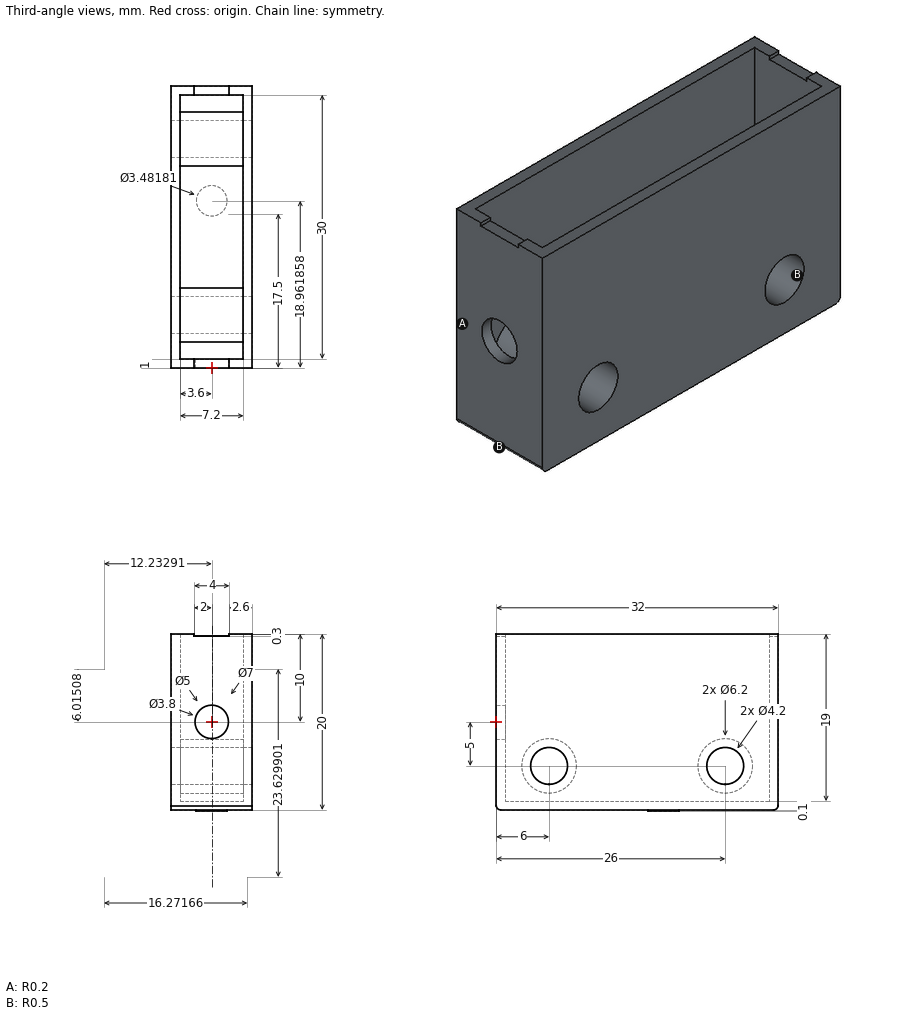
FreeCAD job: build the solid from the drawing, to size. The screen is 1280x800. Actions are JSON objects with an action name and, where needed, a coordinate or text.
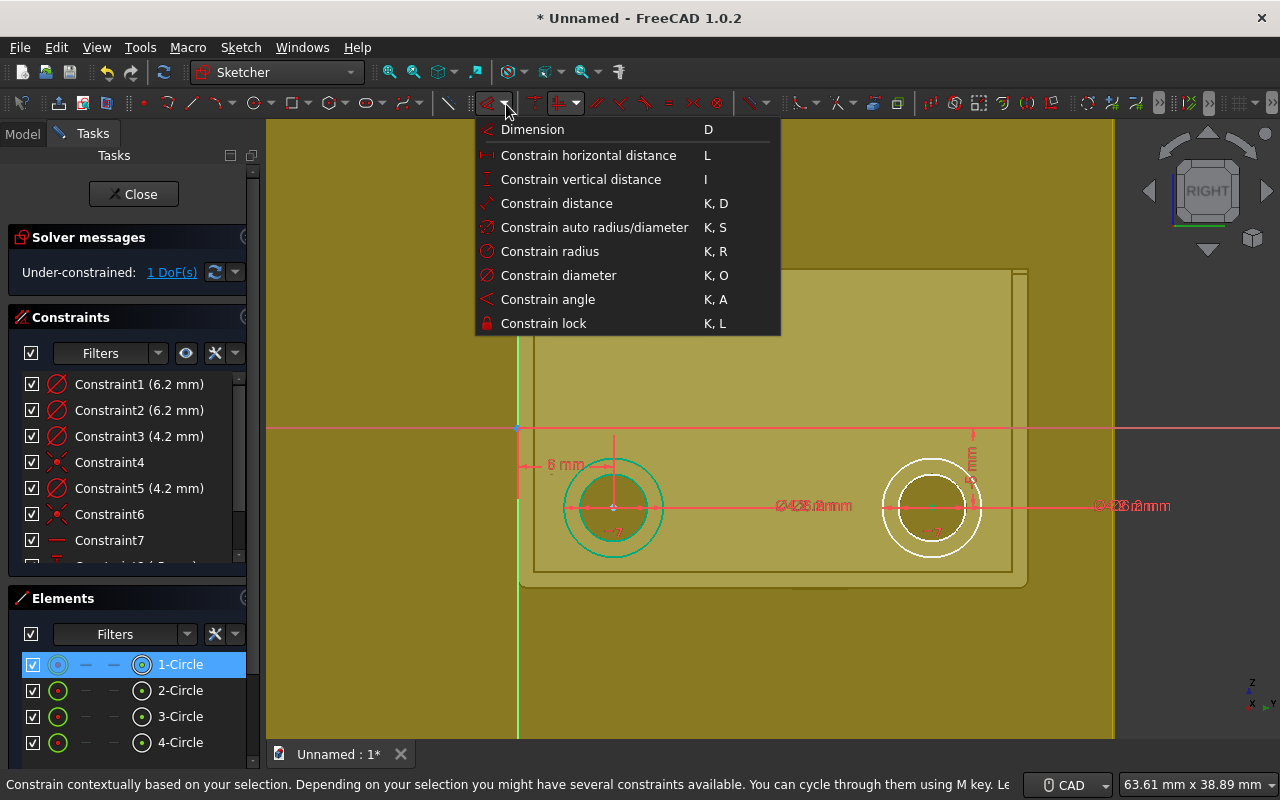
{"action": "left_click", "coordinate": [628, 155]}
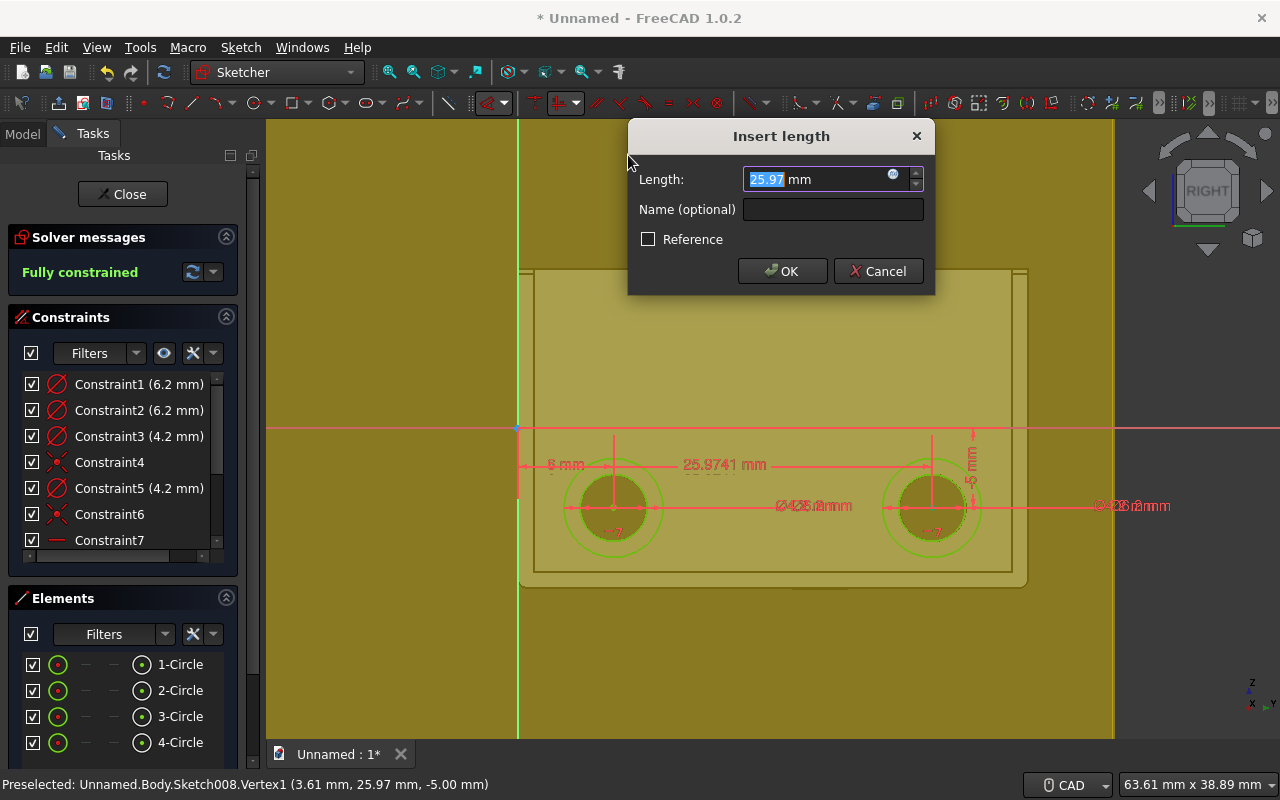
{"action": "type", "text": "26"}
{"action": "key", "text": "Return"}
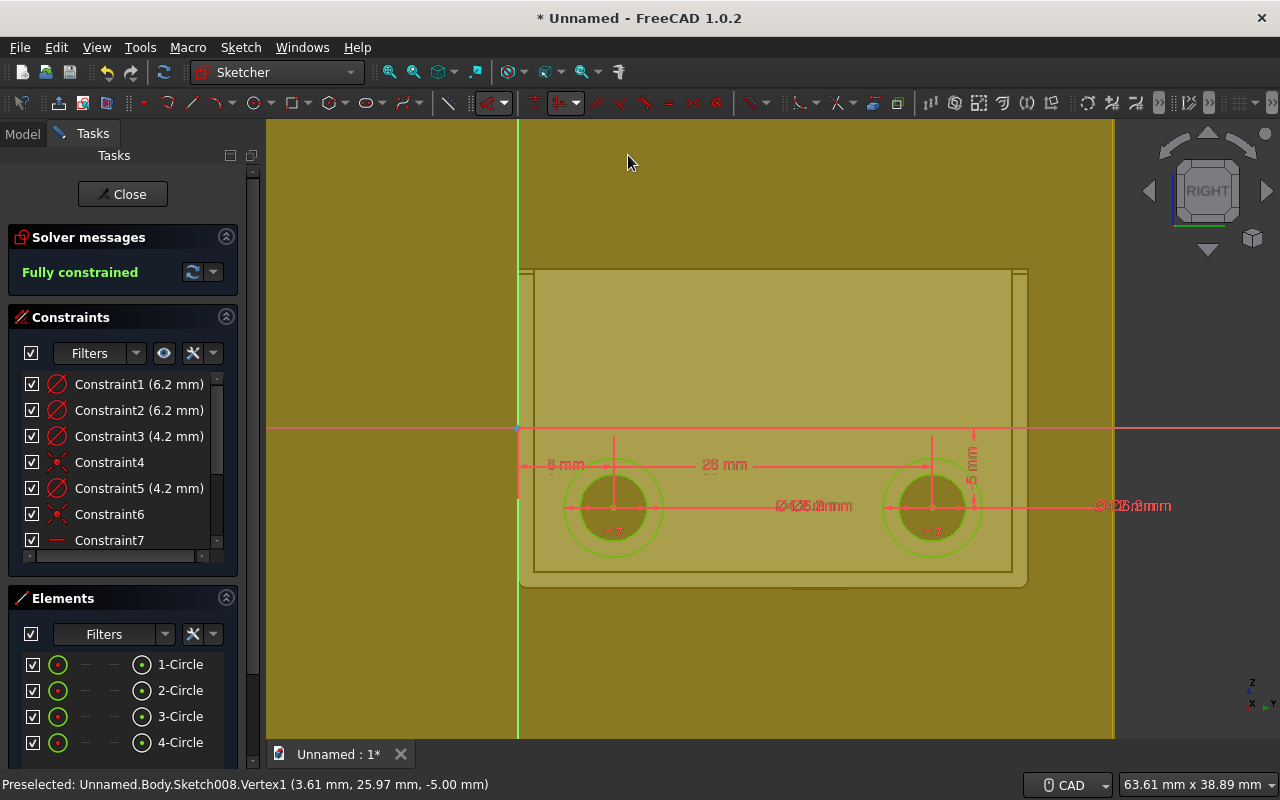
{"action": "left_click", "coordinate": [123, 194]}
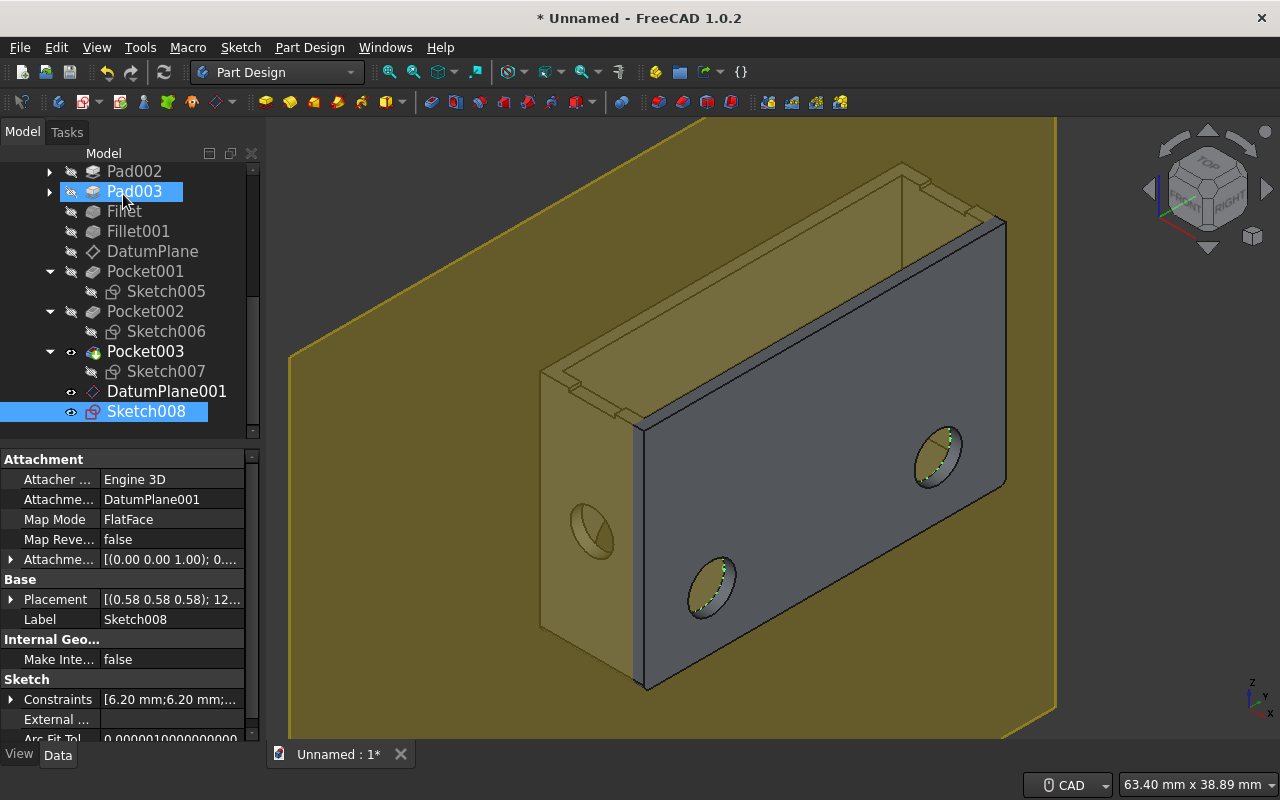
{"action": "left_click", "coordinate": [266, 102]}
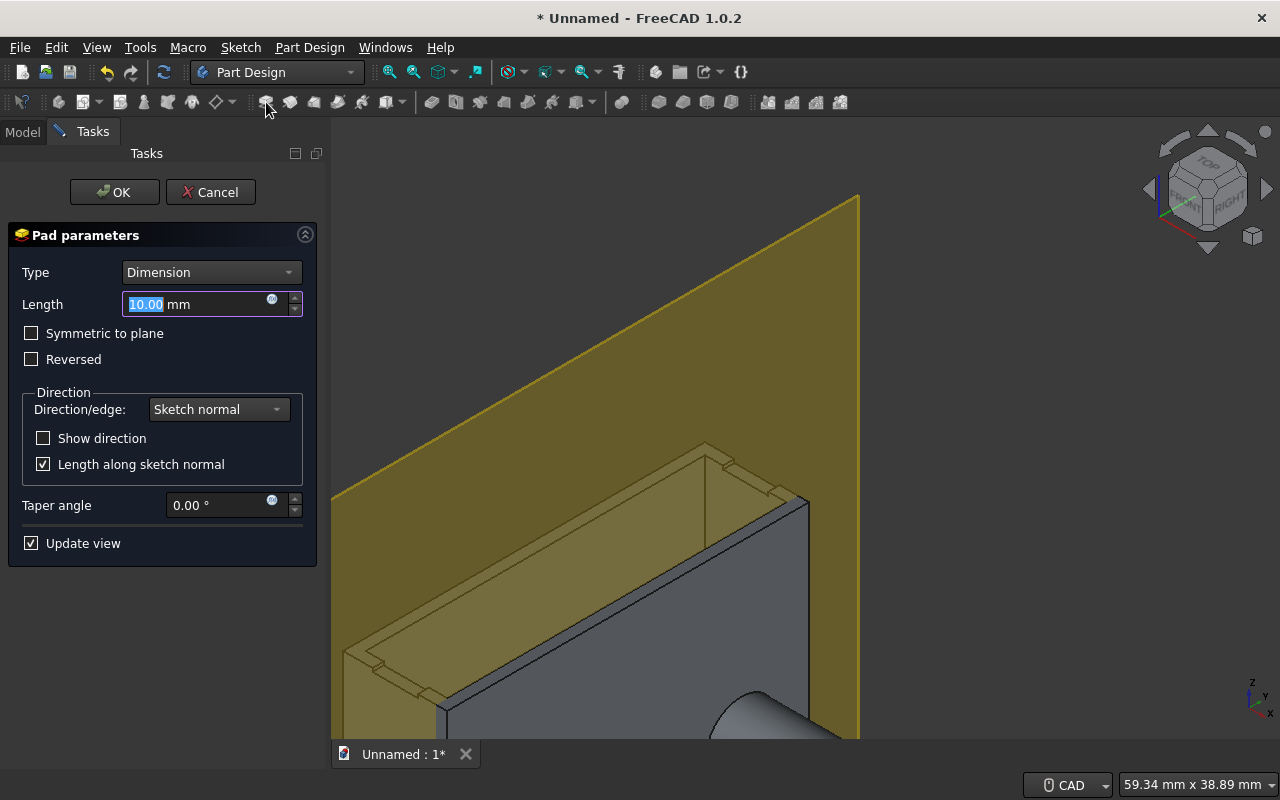
{"action": "type", "text": "7.2"}
{"action": "key", "text": "Tab"}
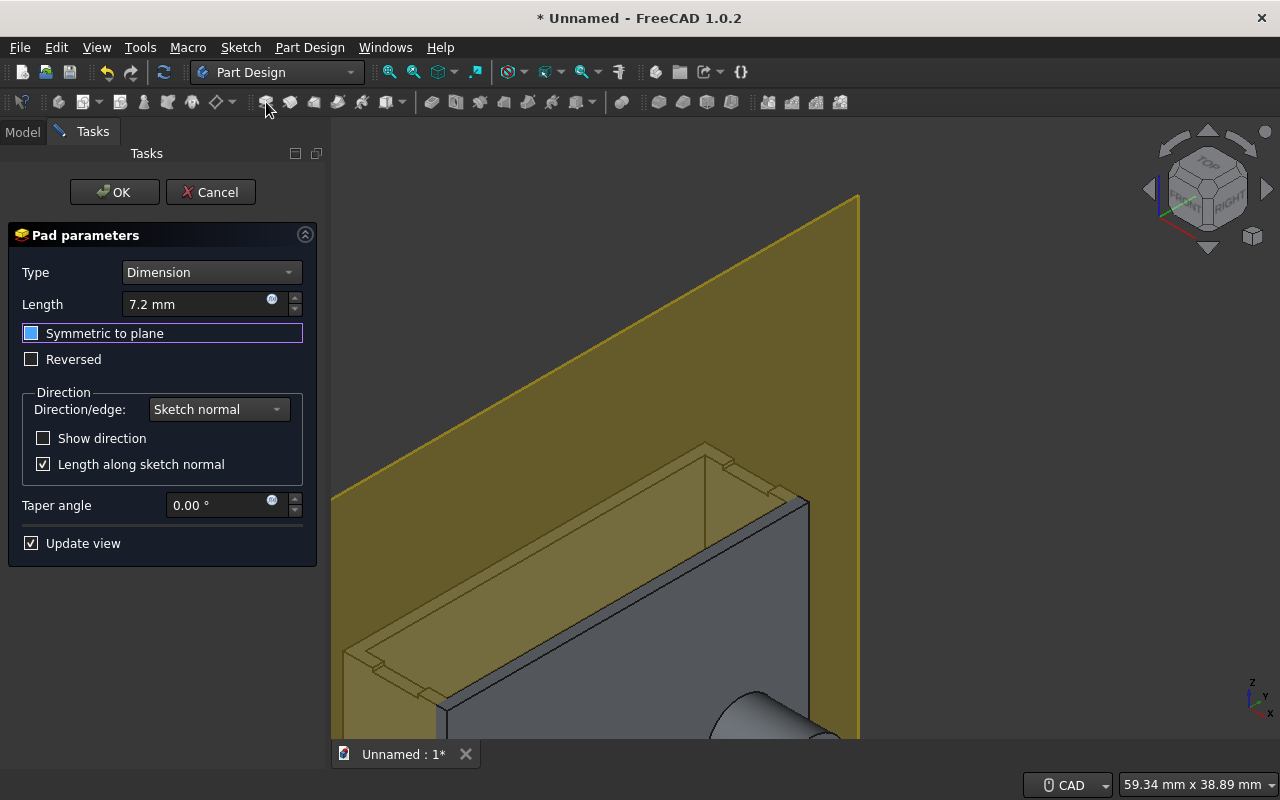
{"action": "left_click", "coordinate": [30, 359]}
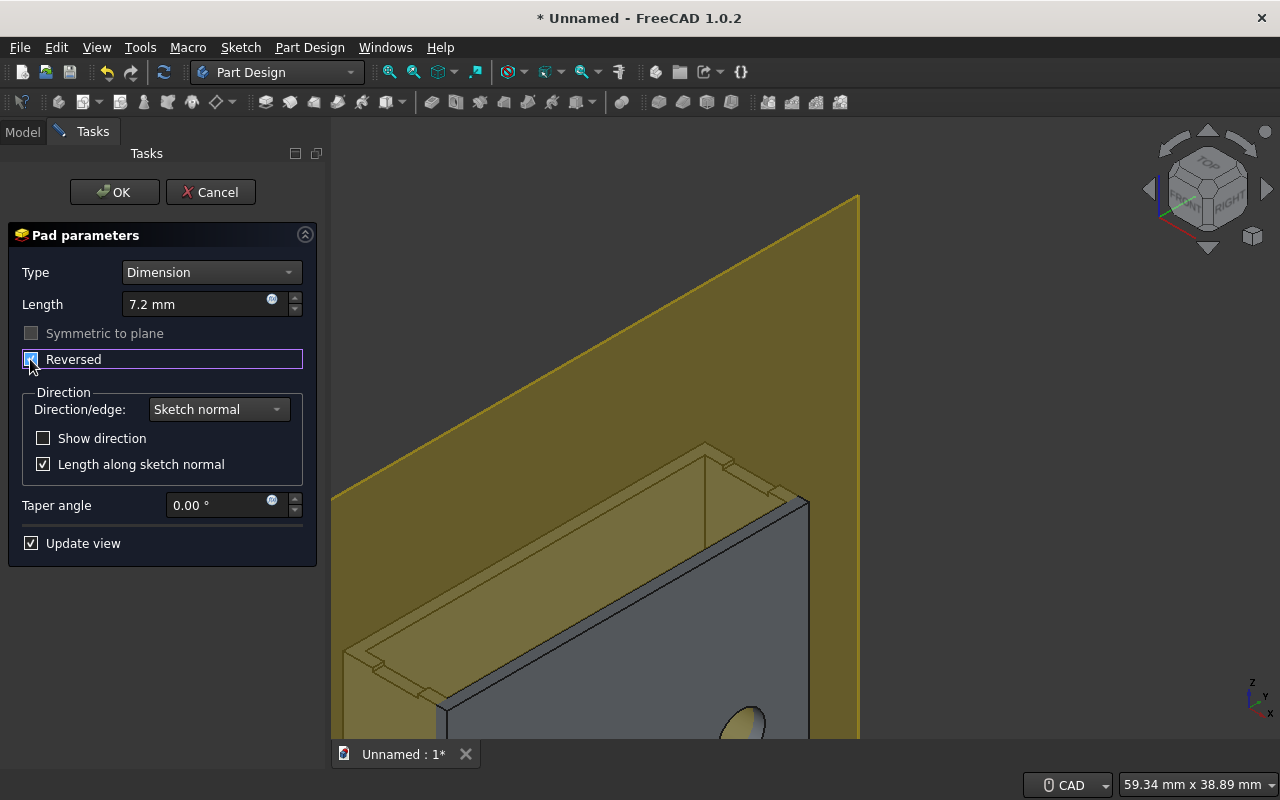
{"action": "left_click", "coordinate": [115, 192]}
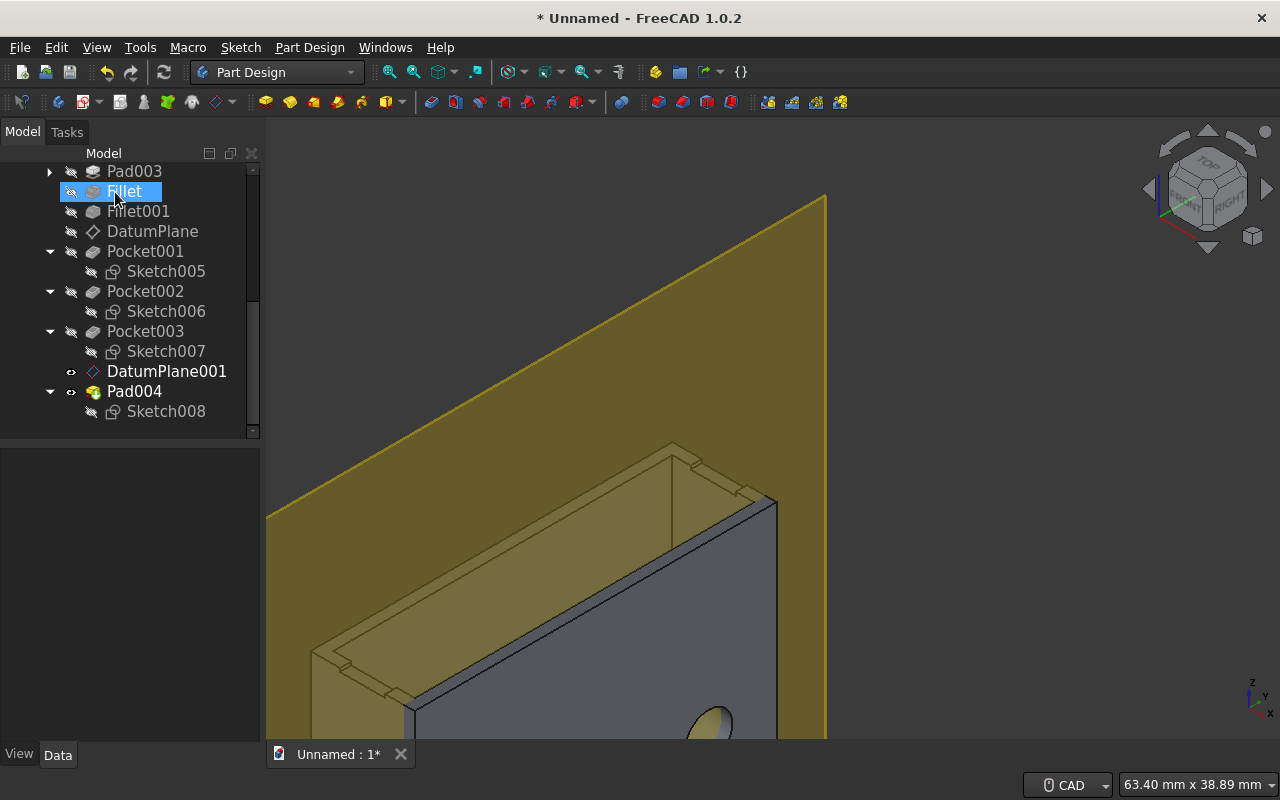
{"action": "left_click", "coordinate": [116, 372]}
{"action": "key", "text": "space"}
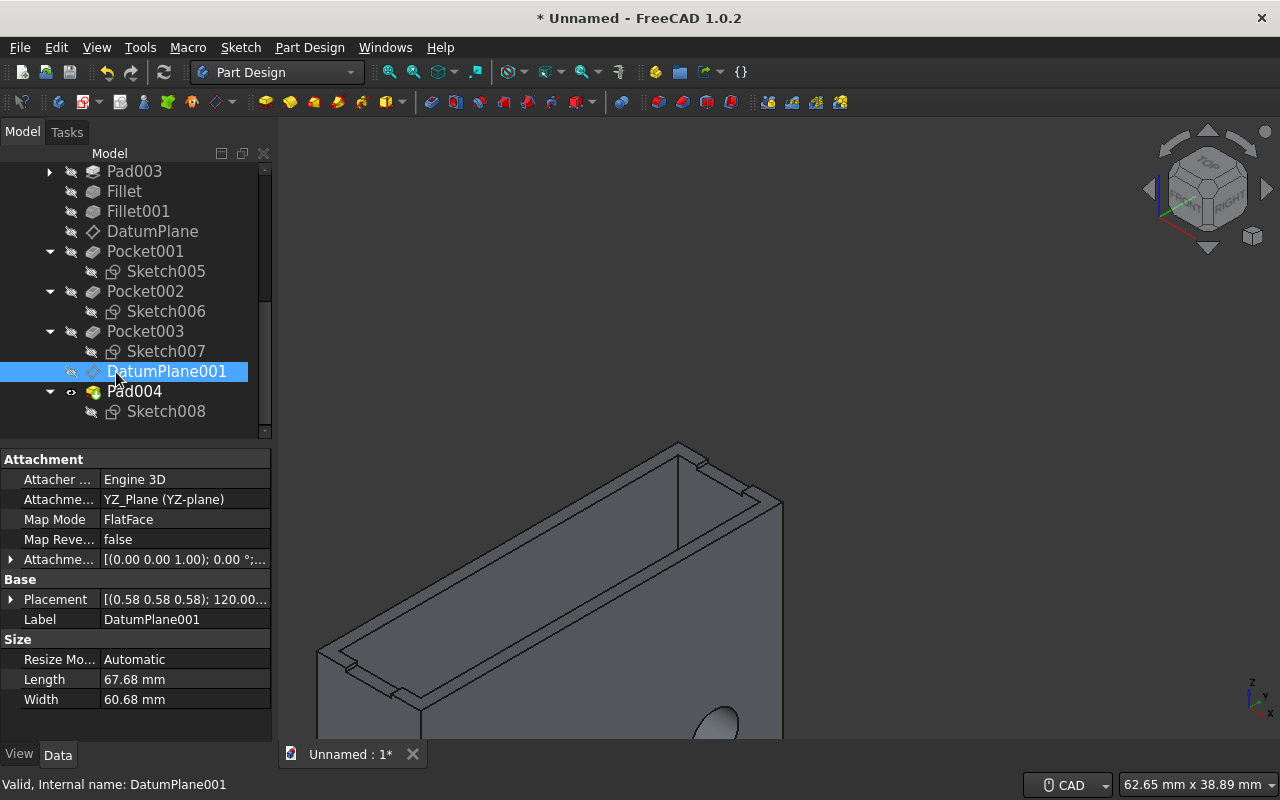
{"action": "left_click", "coordinate": [390, 72]}